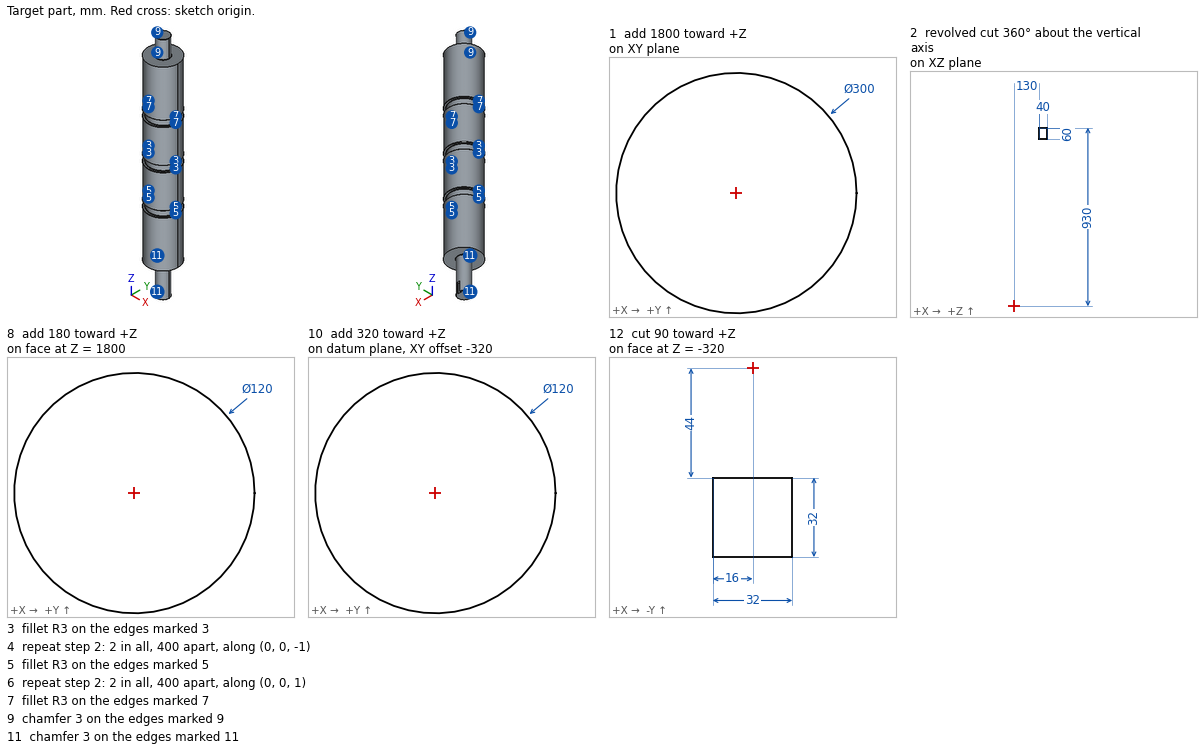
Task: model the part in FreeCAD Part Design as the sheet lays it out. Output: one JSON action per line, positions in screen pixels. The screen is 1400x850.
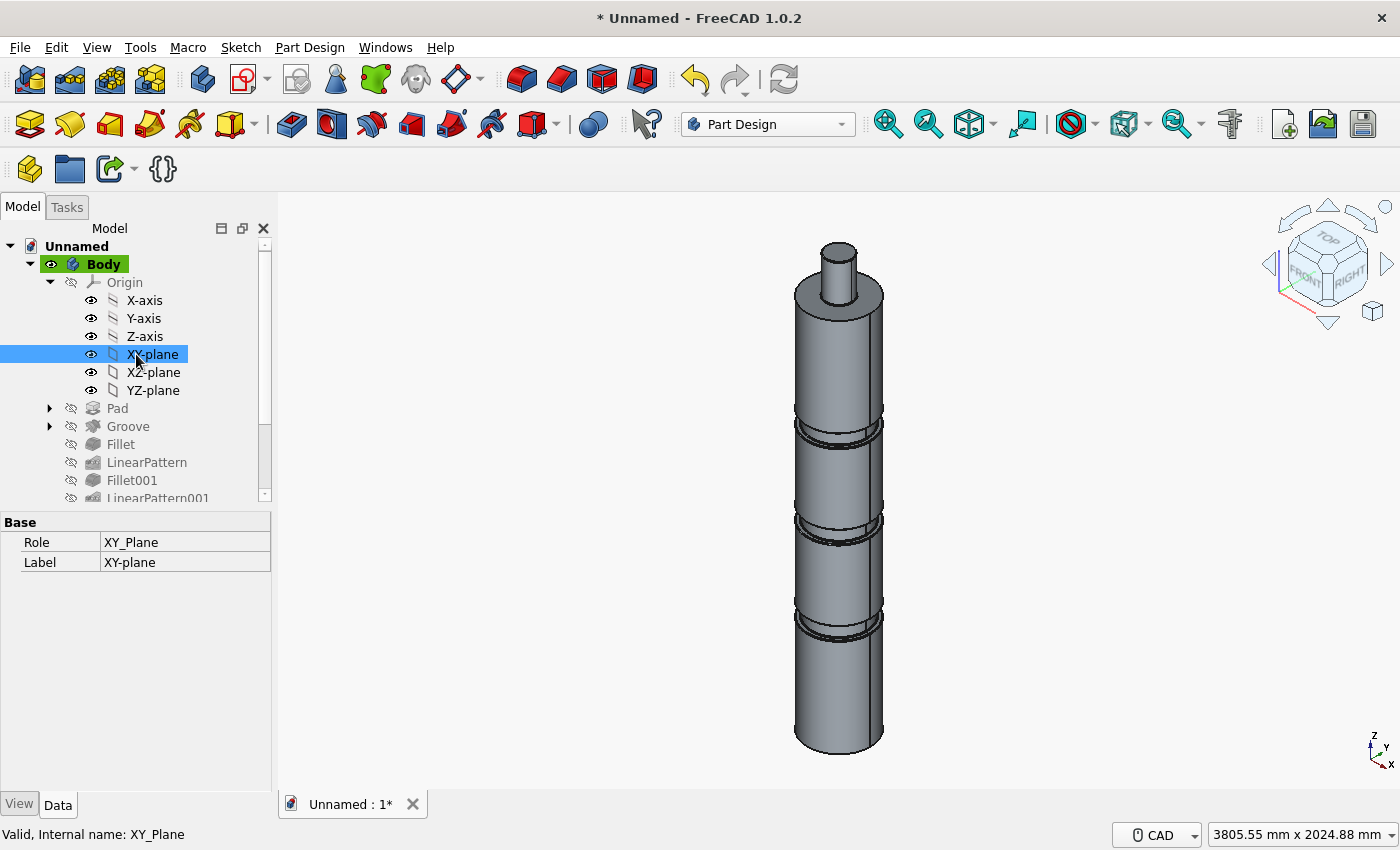
{"action": "left_click", "coordinate": [456, 80]}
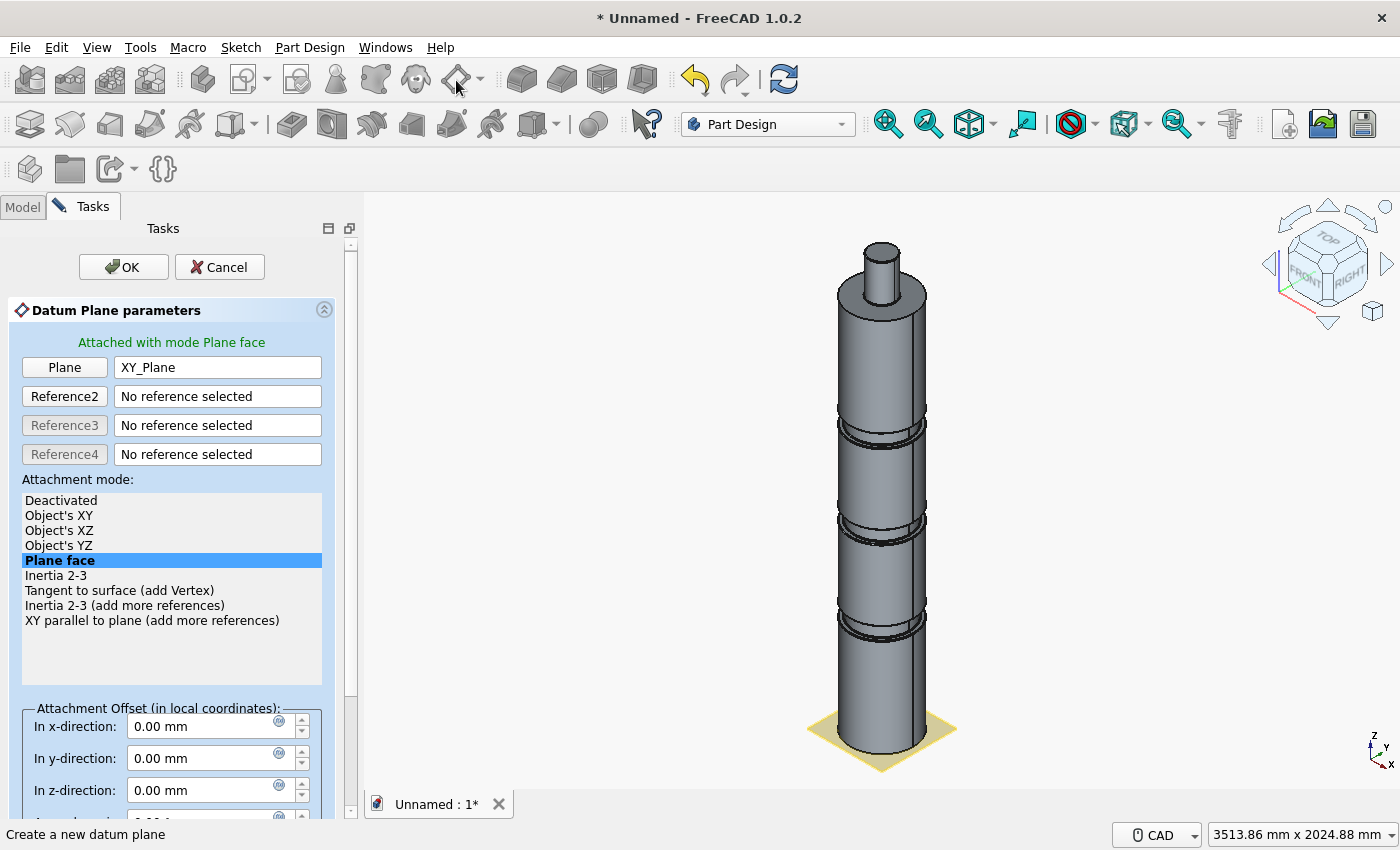
{"action": "triple_click", "coordinate": [210, 790]}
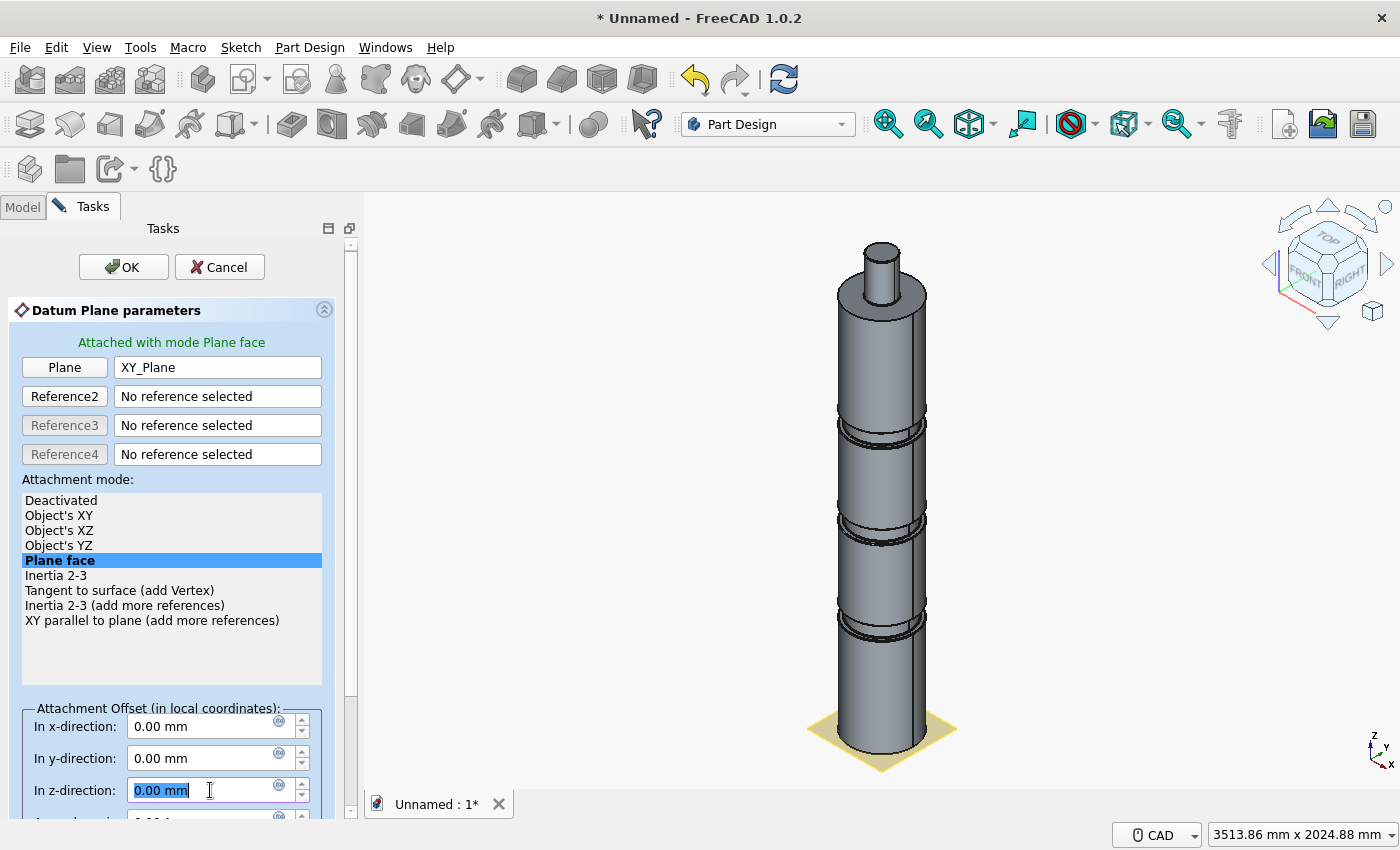
{"action": "type", "text": "-320"}
{"action": "key", "text": "Tab"}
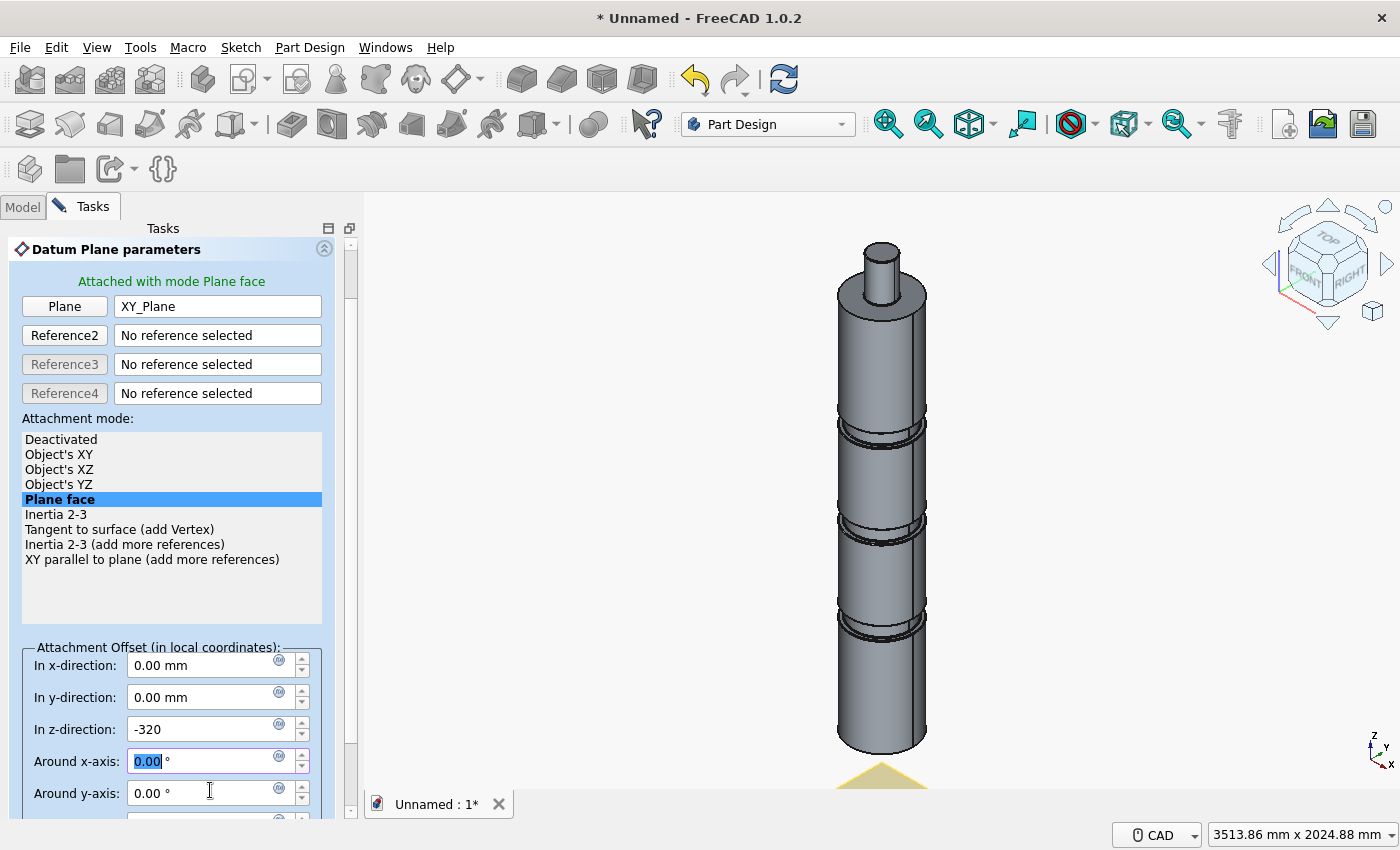
{"action": "scroll", "coordinate": [351, 528], "scroll_direction": "up", "scroll_amount": 2}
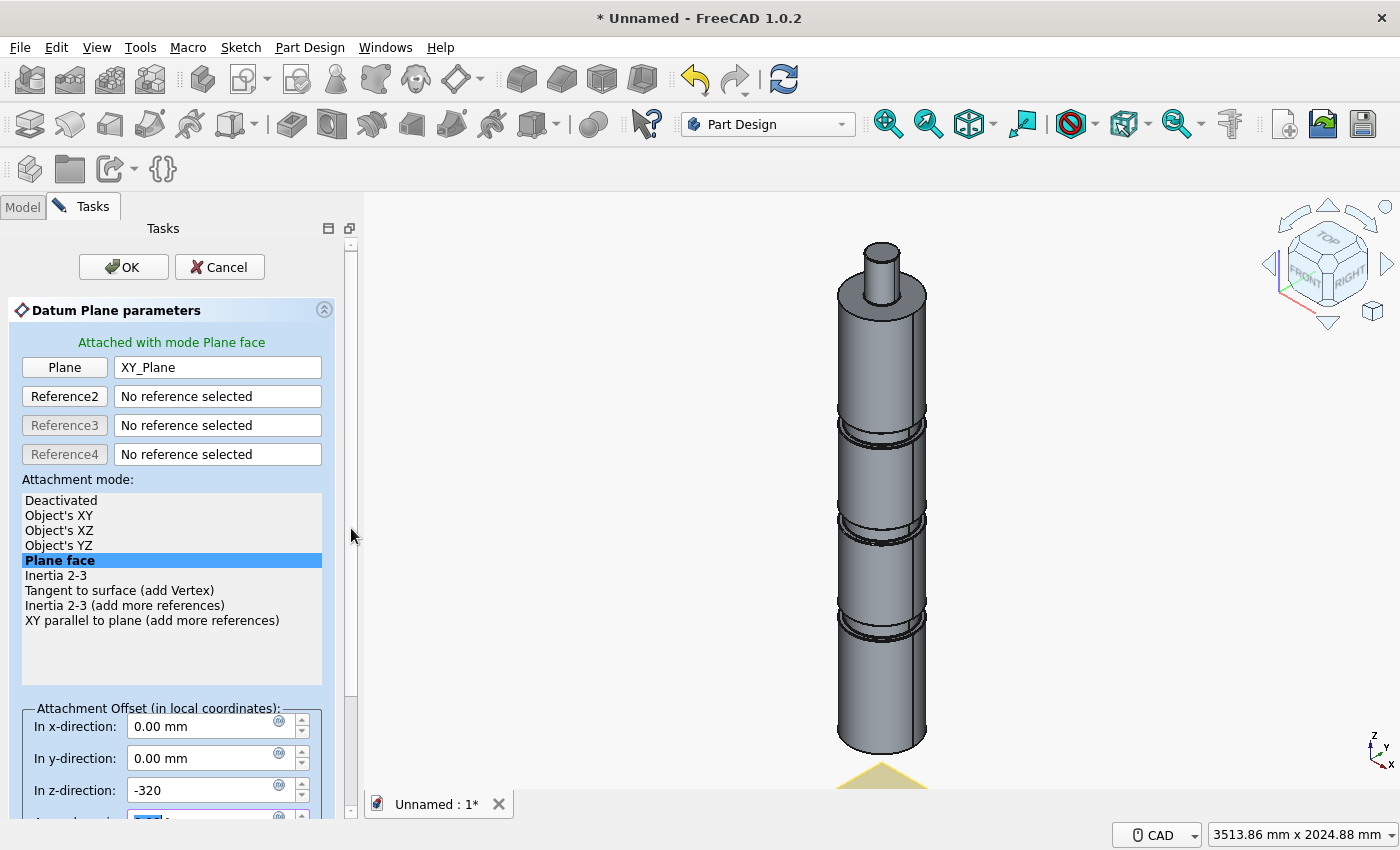
{"action": "left_click", "coordinate": [124, 267]}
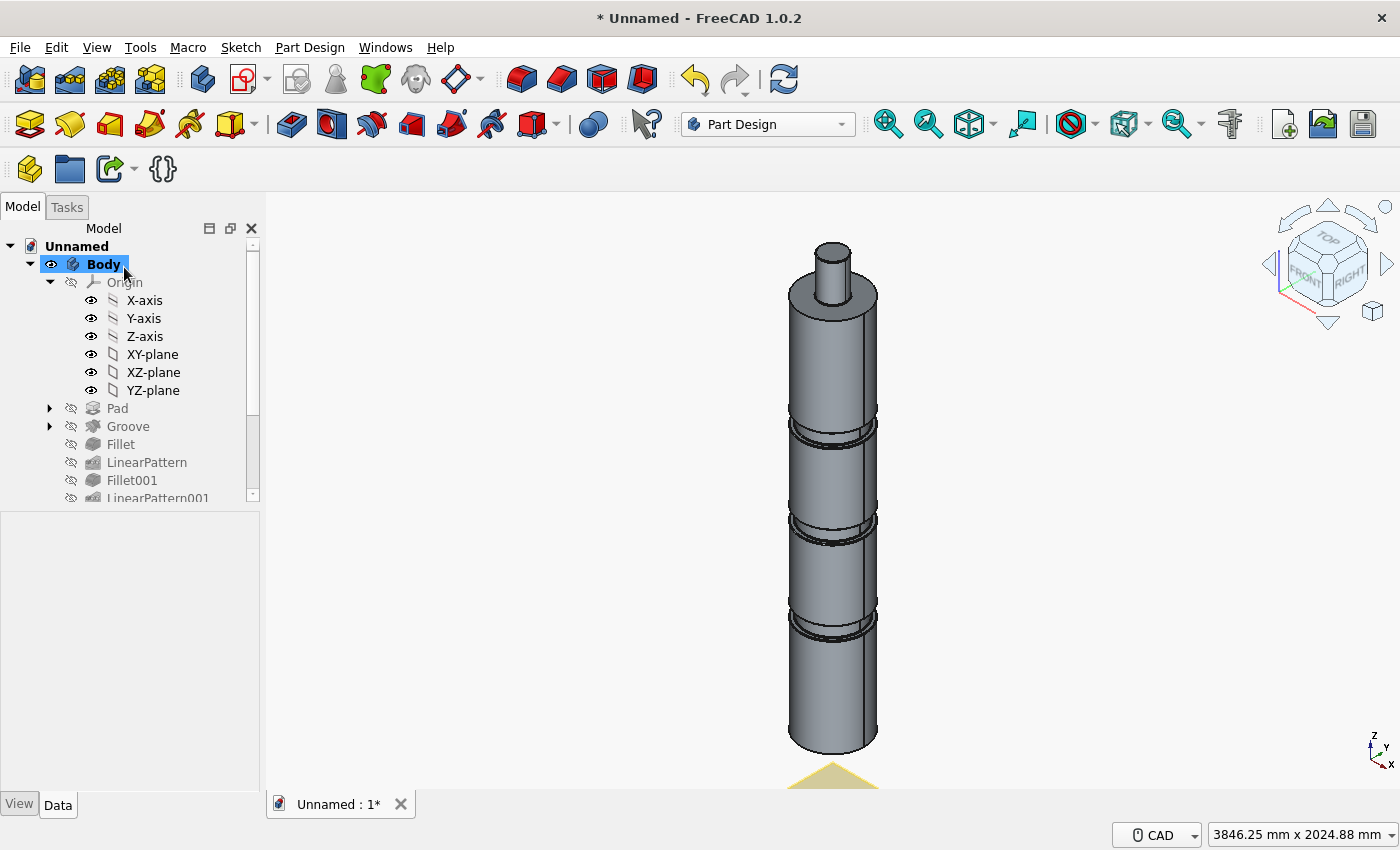
{"action": "scroll", "coordinate": [100, 368], "scroll_direction": "down", "scroll_amount": 3}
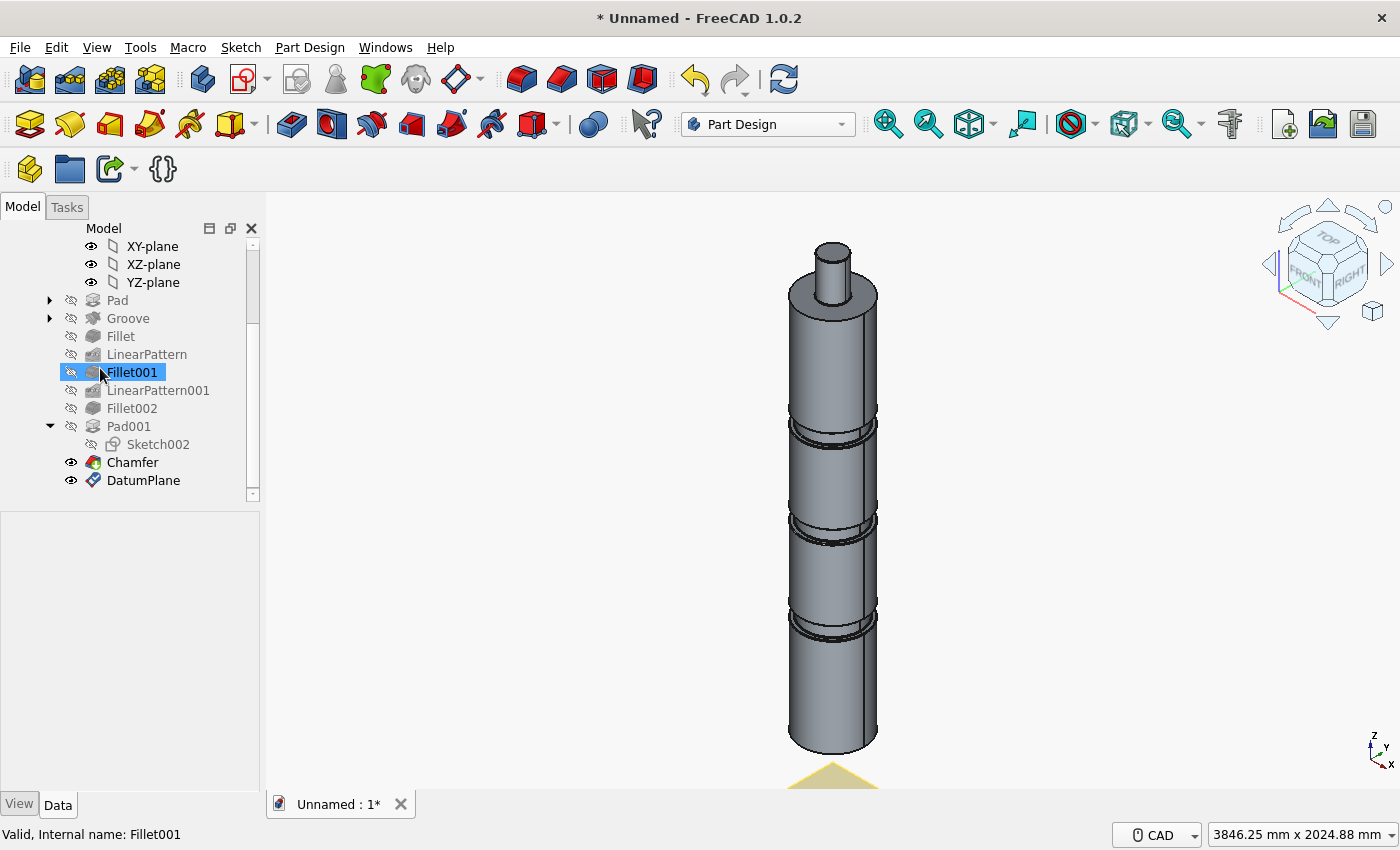
{"action": "left_click", "coordinate": [116, 480]}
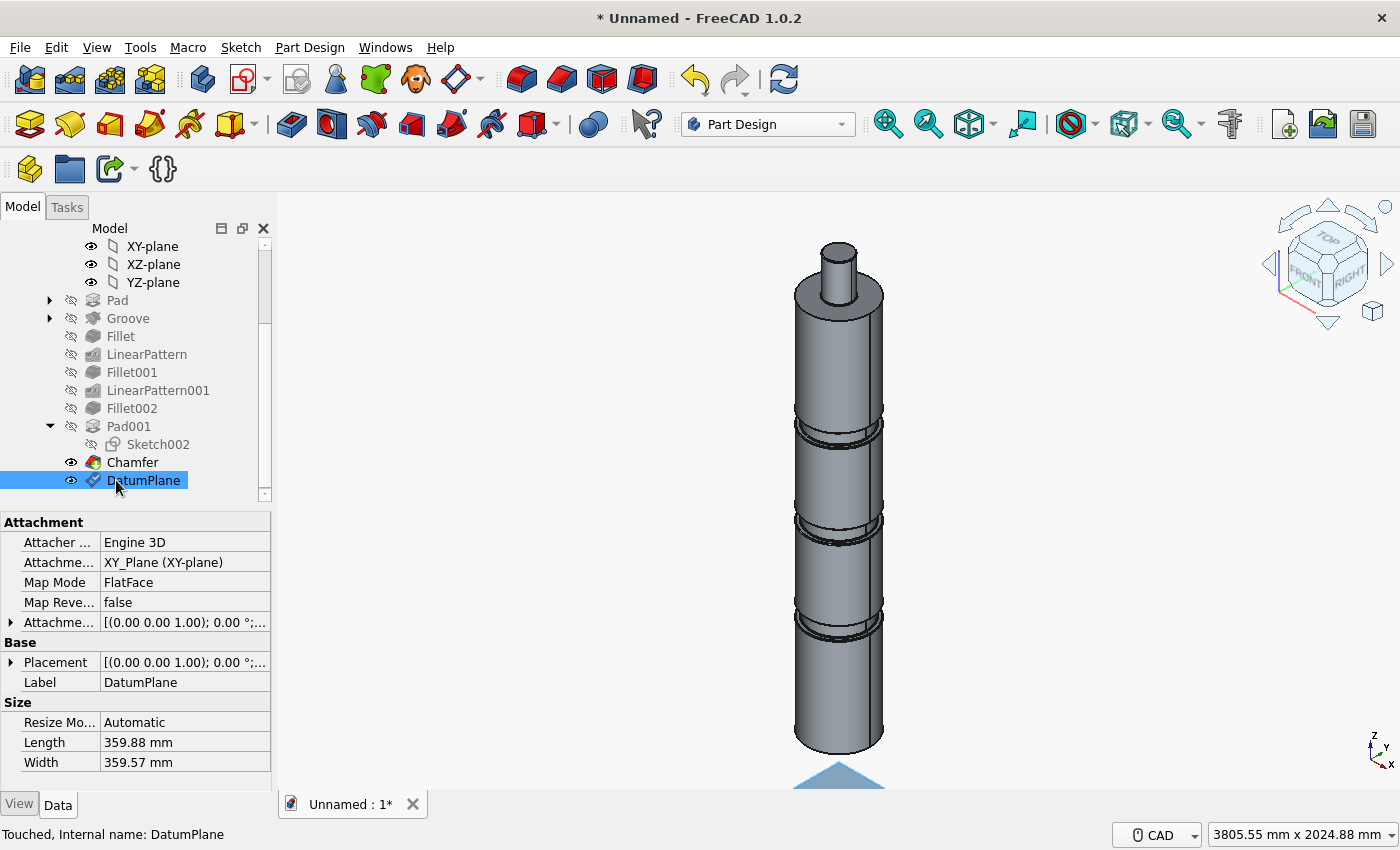
{"action": "left_click", "coordinate": [244, 80]}